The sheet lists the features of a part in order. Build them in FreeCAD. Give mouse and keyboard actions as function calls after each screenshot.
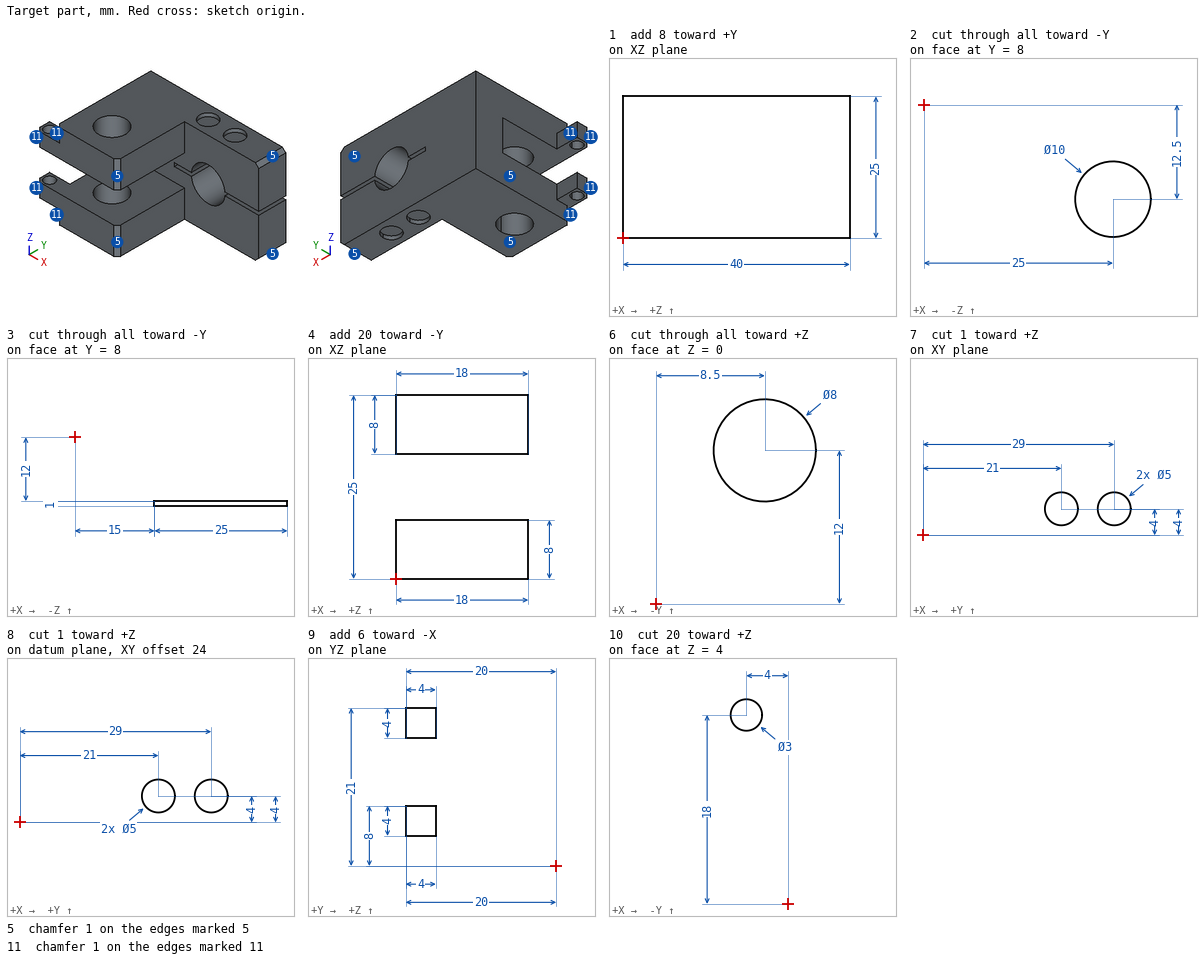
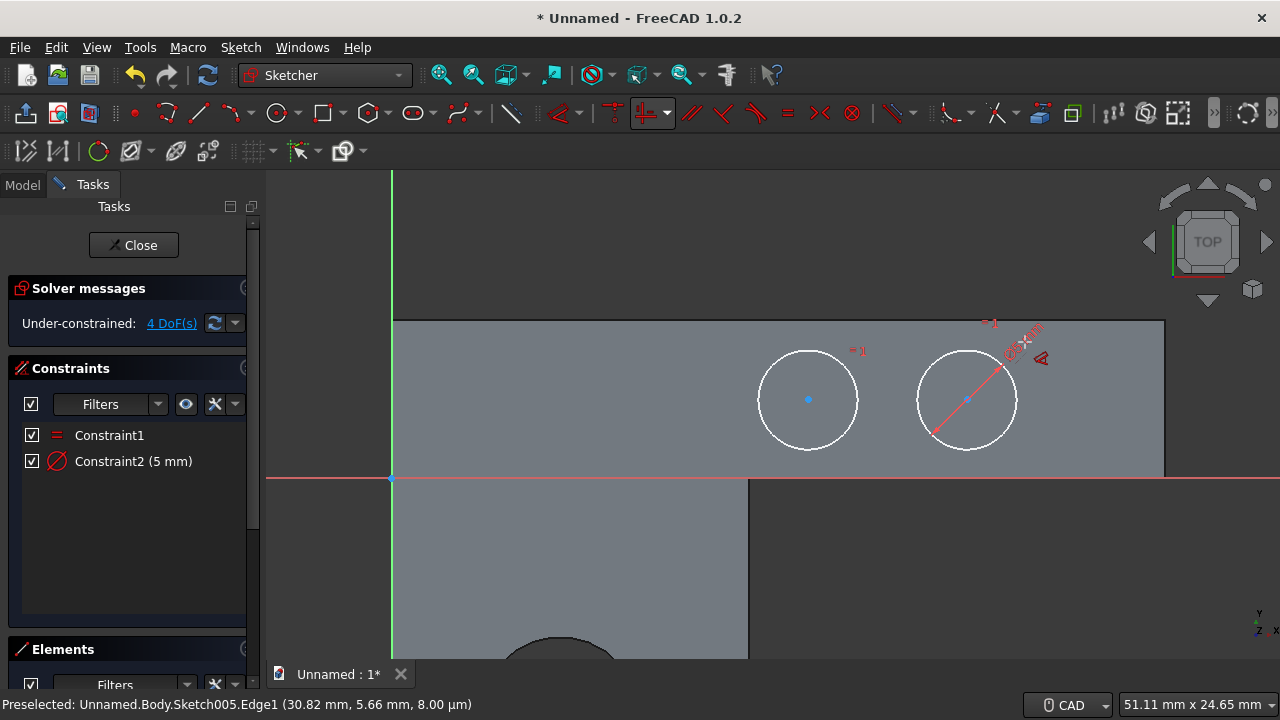
click(967, 400)
click(358, 439)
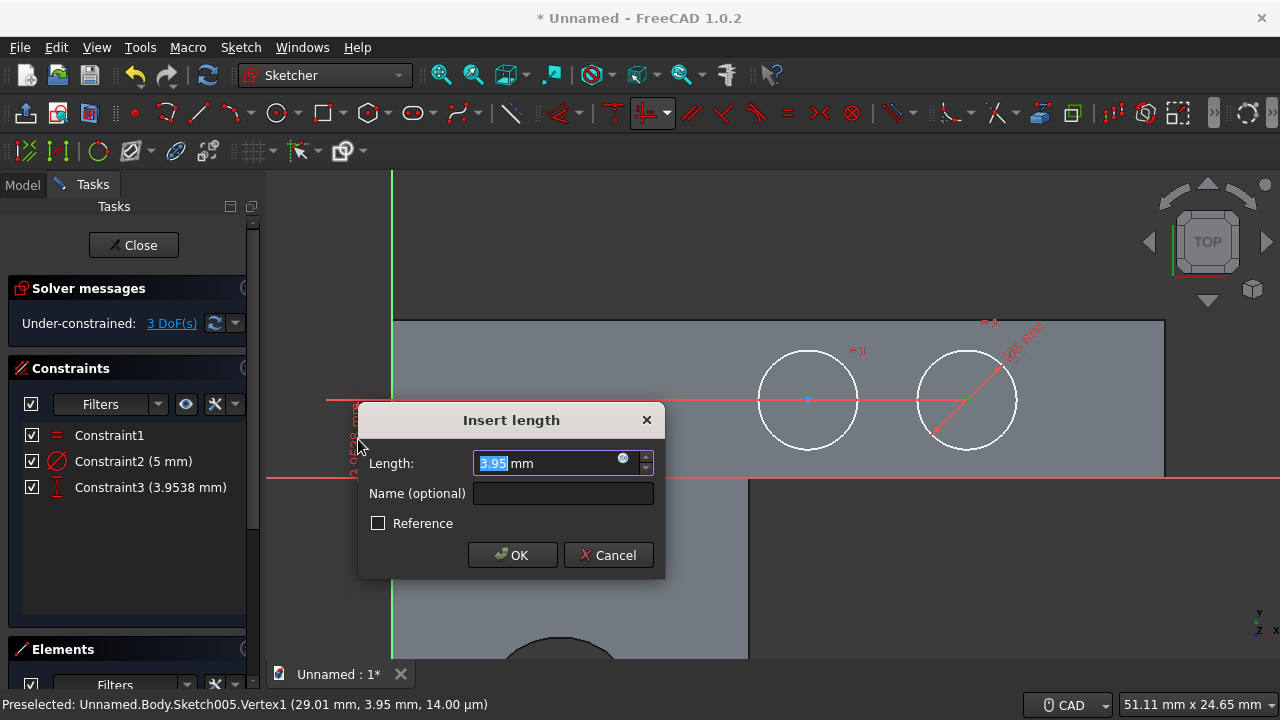
text(4)
key(Return)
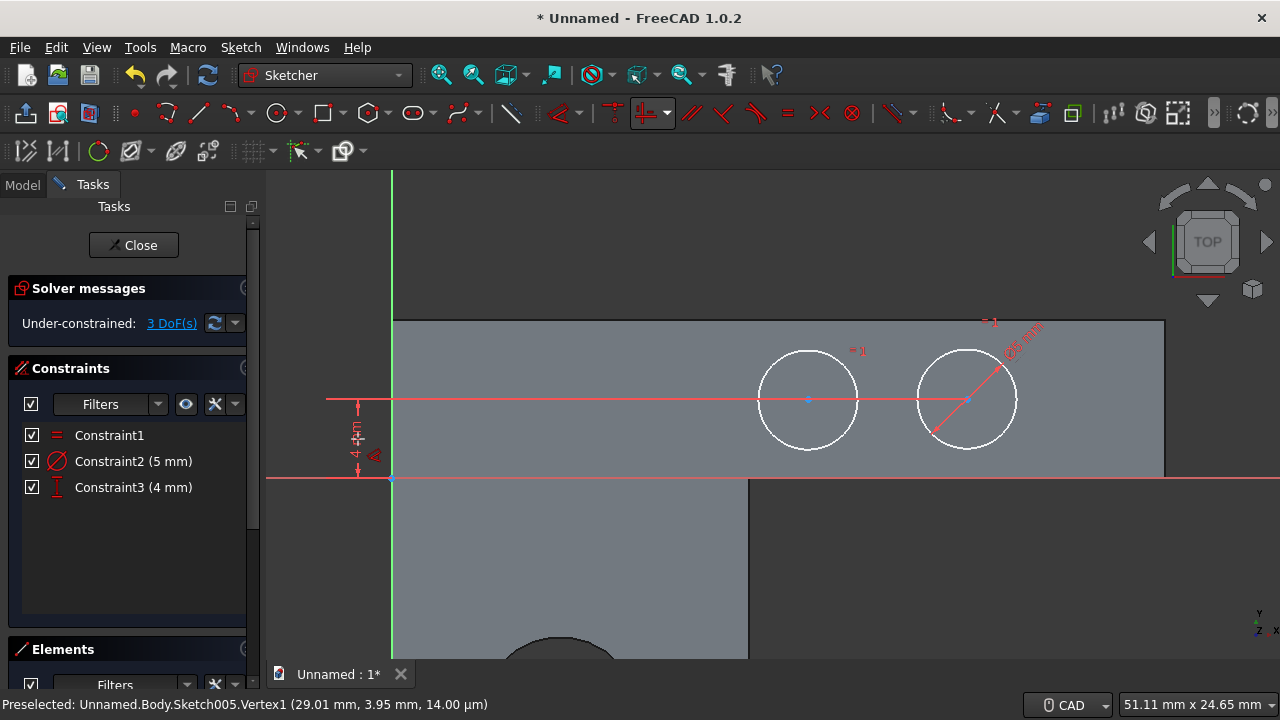
click(808, 400)
click(358, 412)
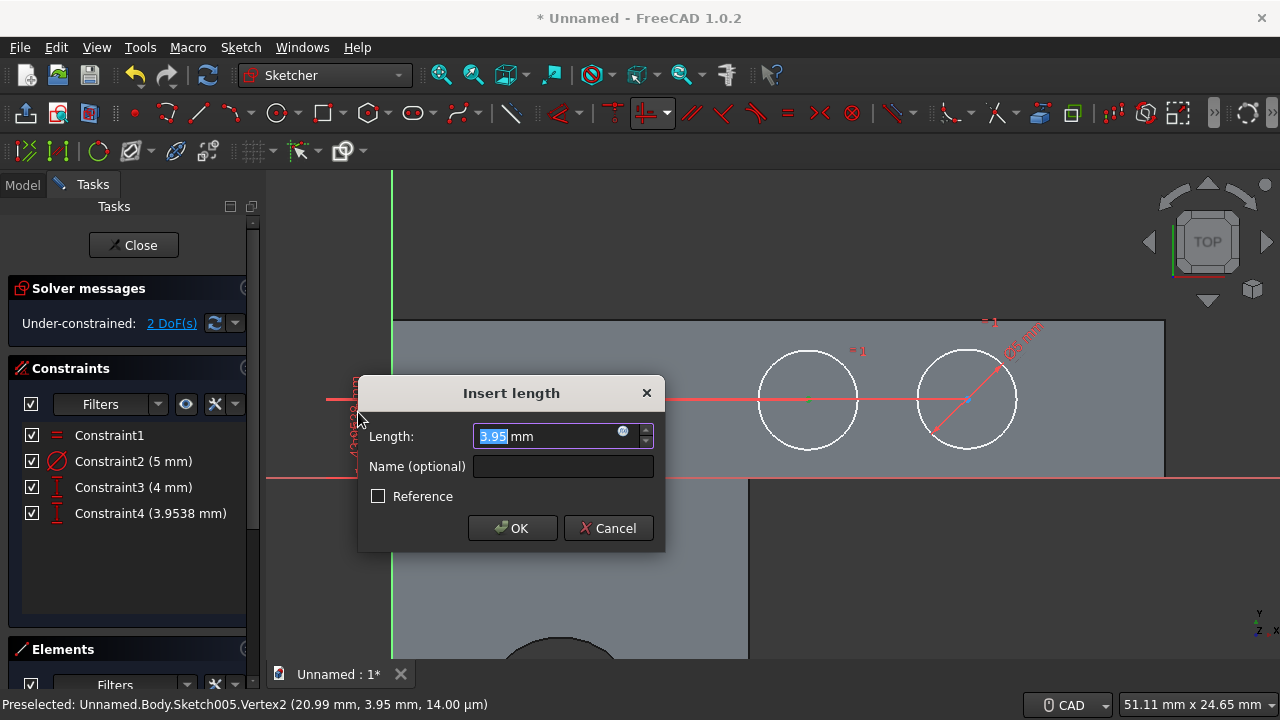
text(4)
key(Return)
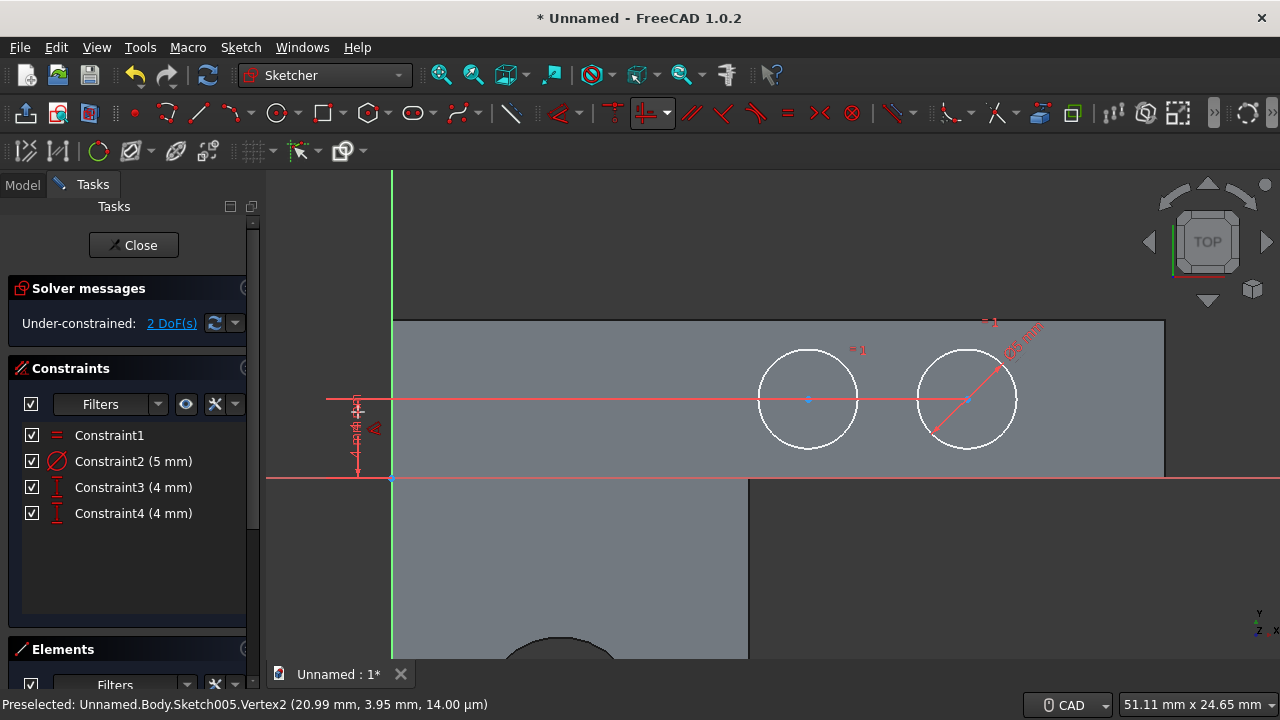
click(967, 399)
click(679, 512)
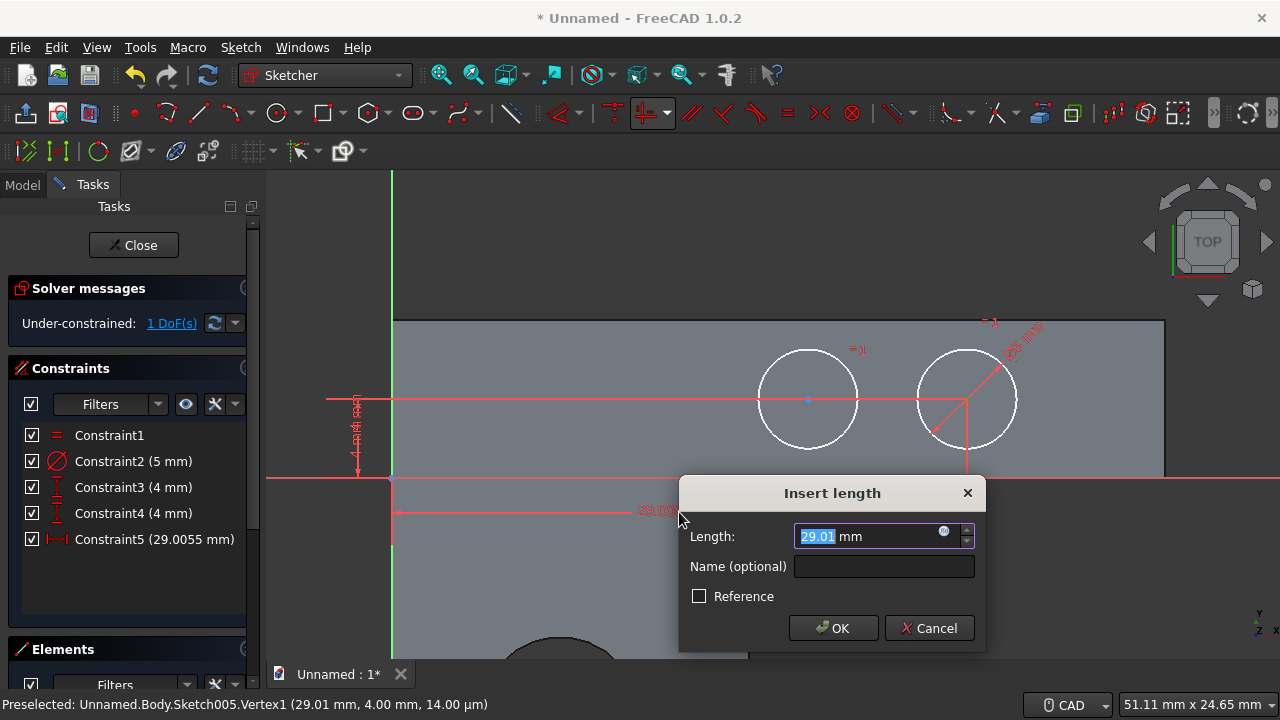
text(29)
key(Return)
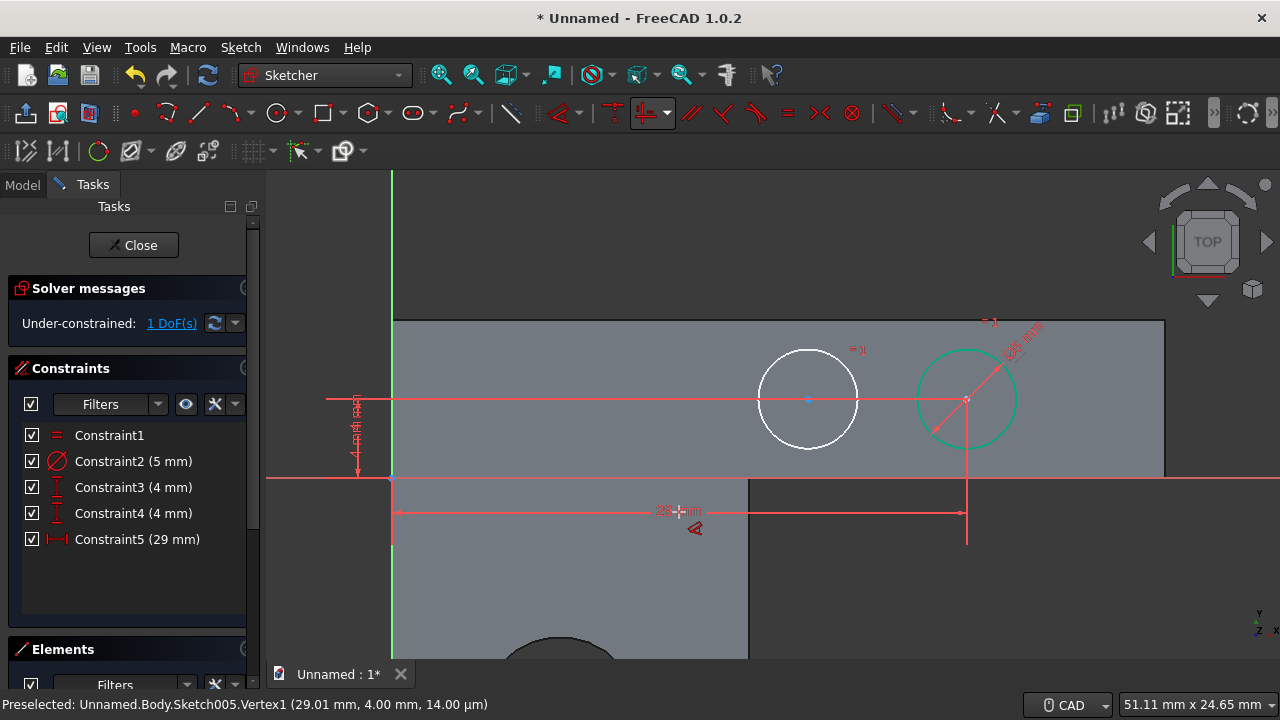
click(808, 399)
click(600, 512)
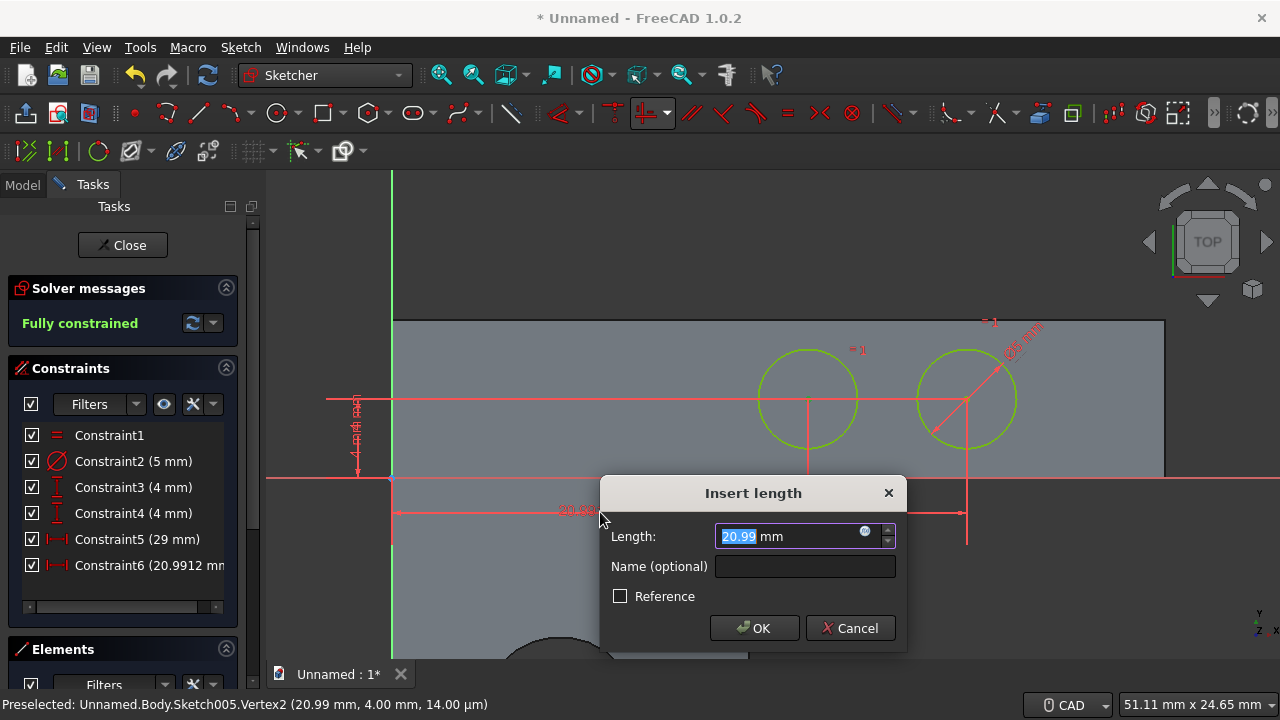
text(21)
key(Return)
key(Escape)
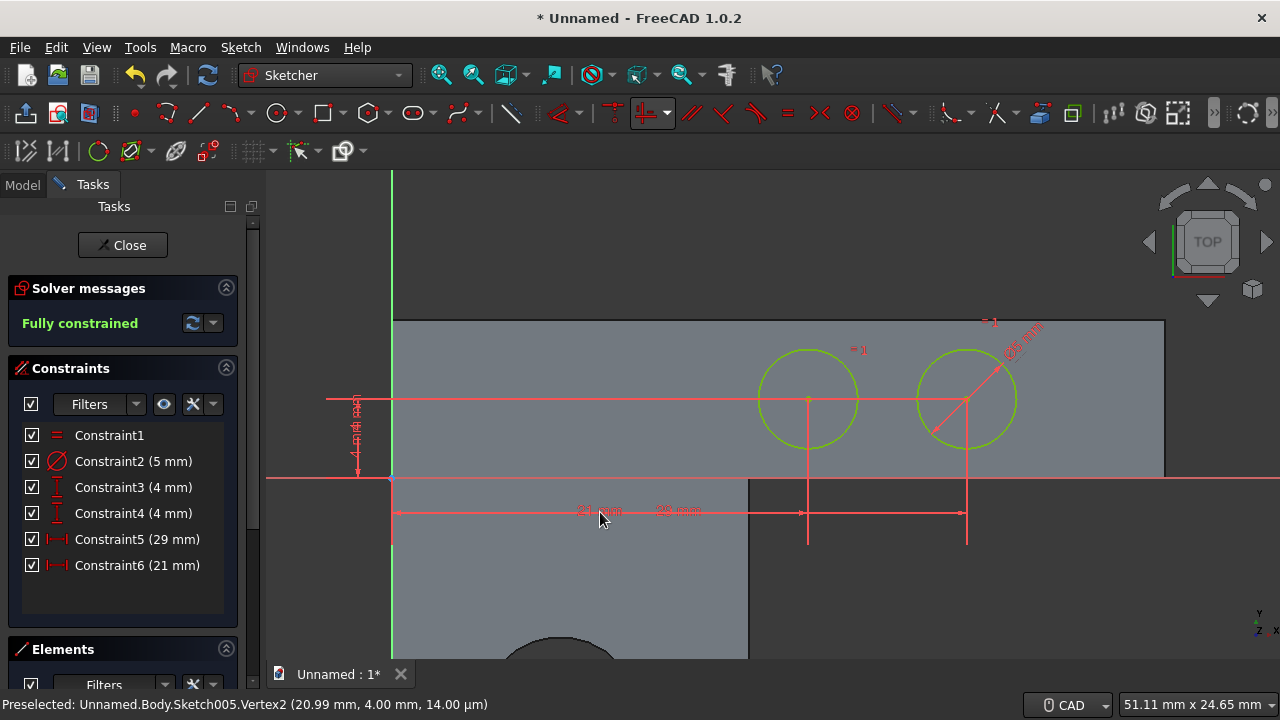
click(123, 245)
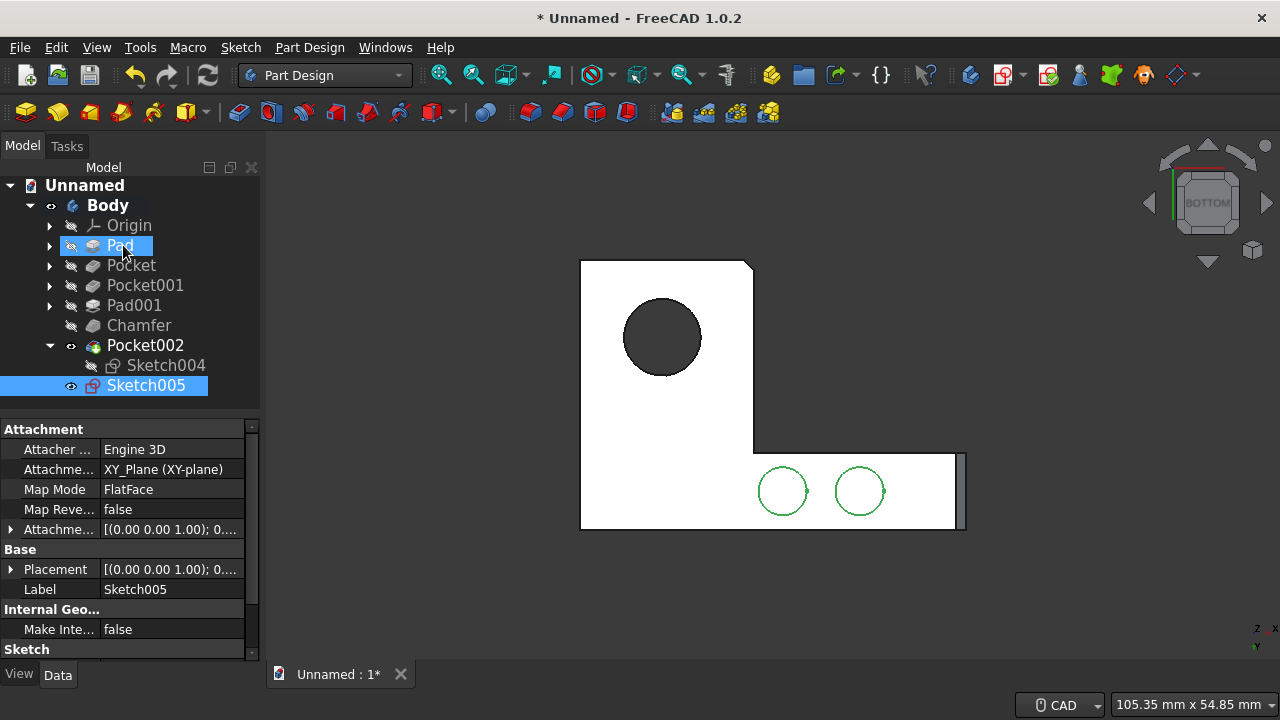
click(240, 112)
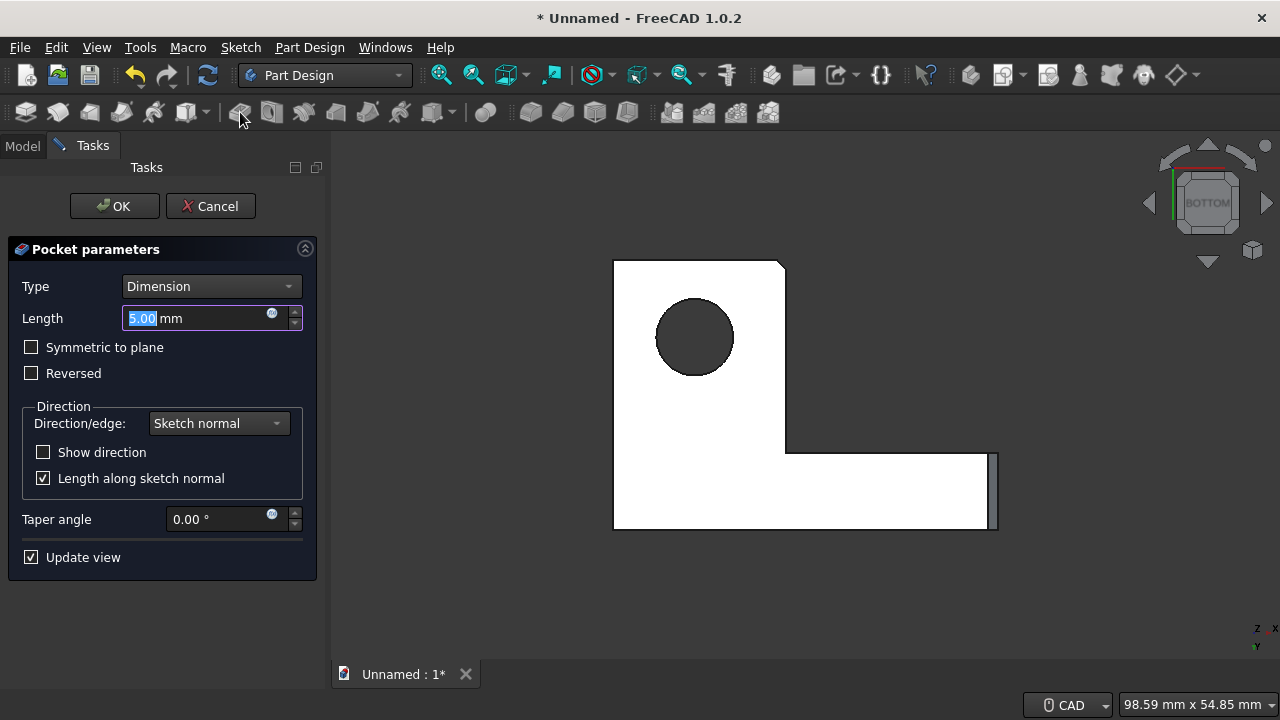
text(1)
key(Tab)